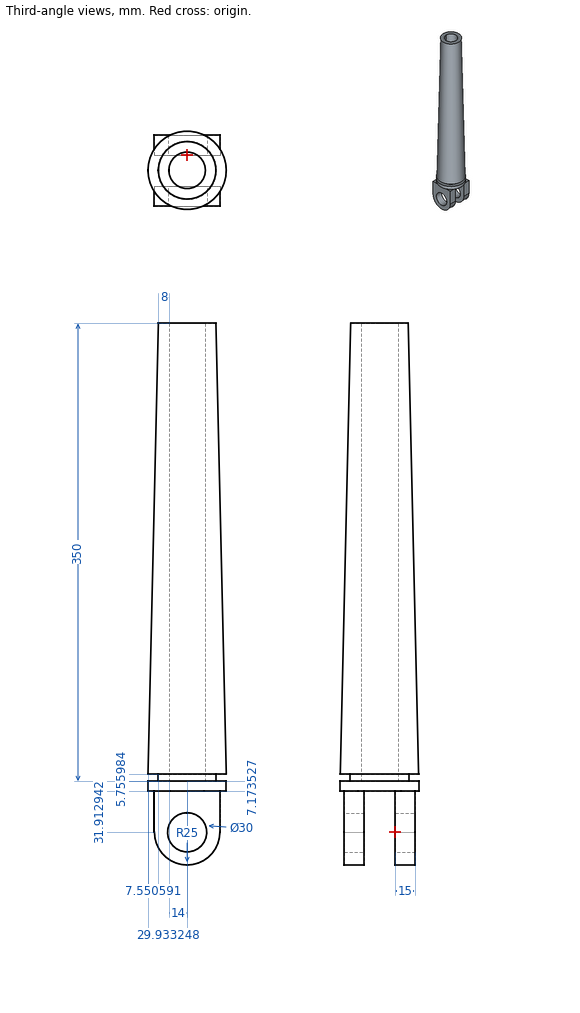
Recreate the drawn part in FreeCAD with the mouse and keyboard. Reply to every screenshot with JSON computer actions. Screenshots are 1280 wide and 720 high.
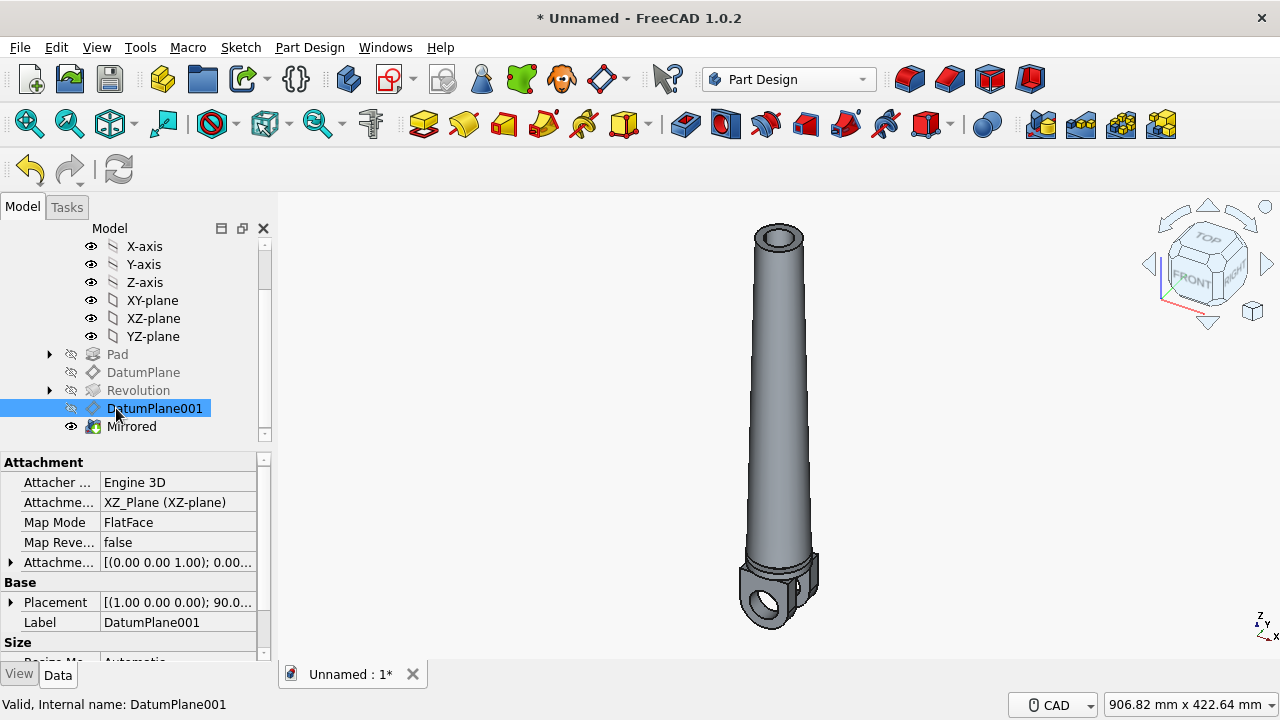
{"action": "key", "text": "0"}